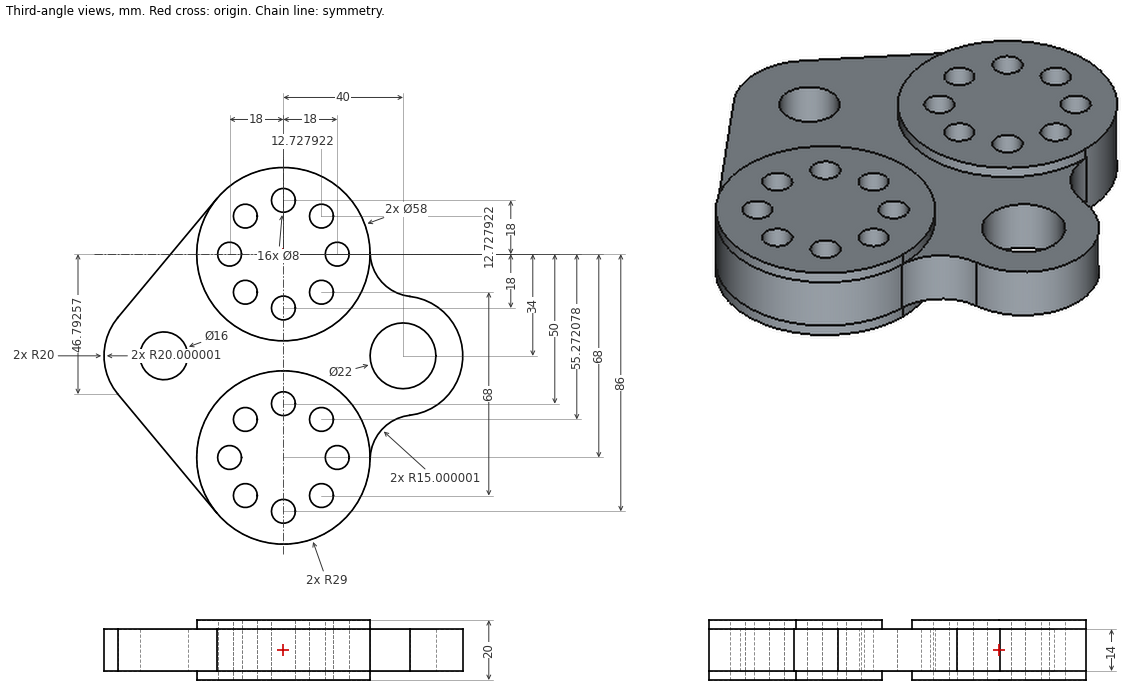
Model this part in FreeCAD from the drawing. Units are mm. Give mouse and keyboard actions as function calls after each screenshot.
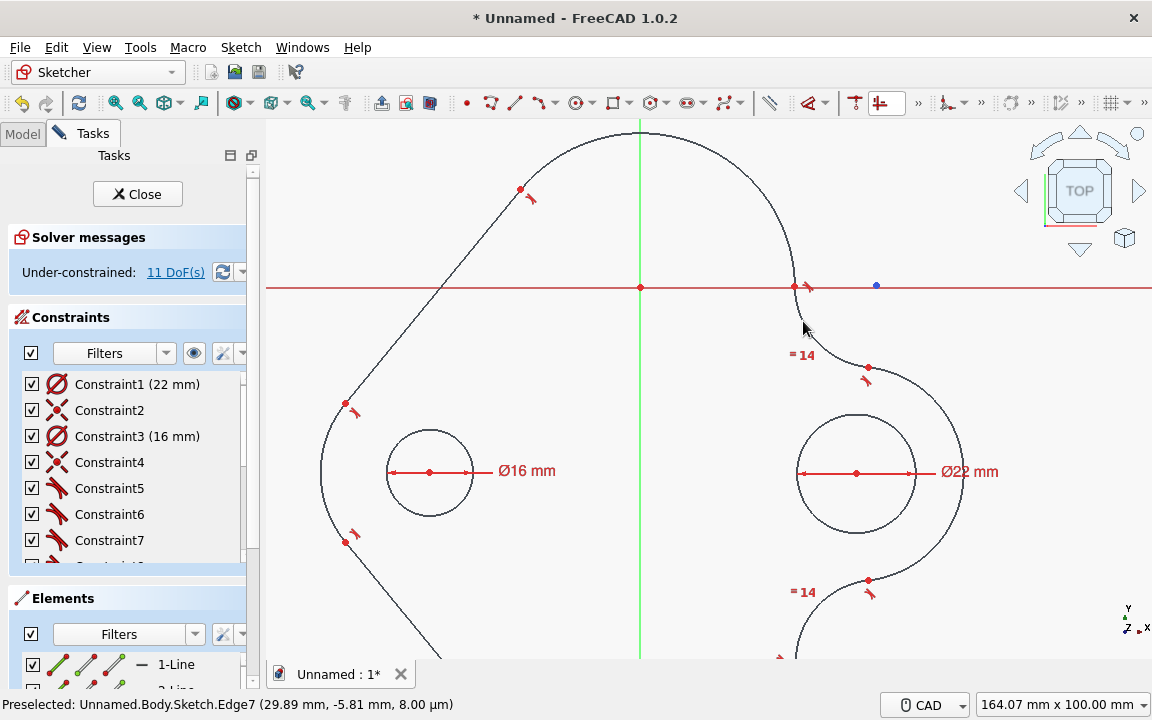
scroll(641, 289, down, 3)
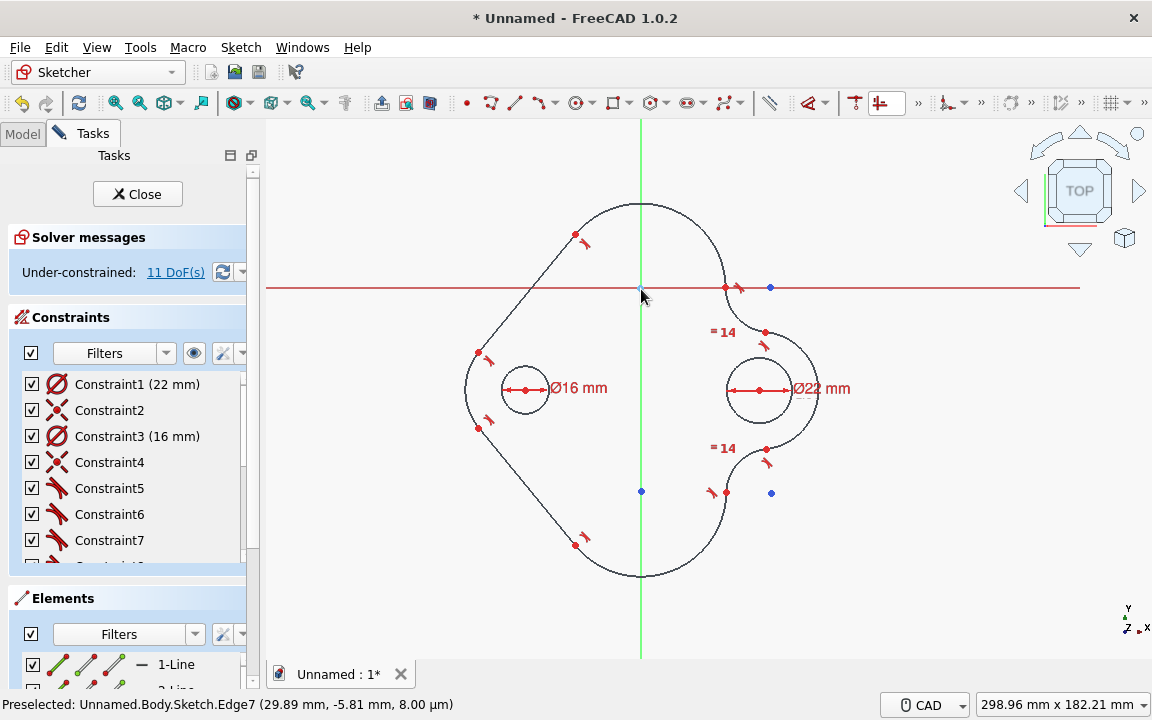
click(628, 576)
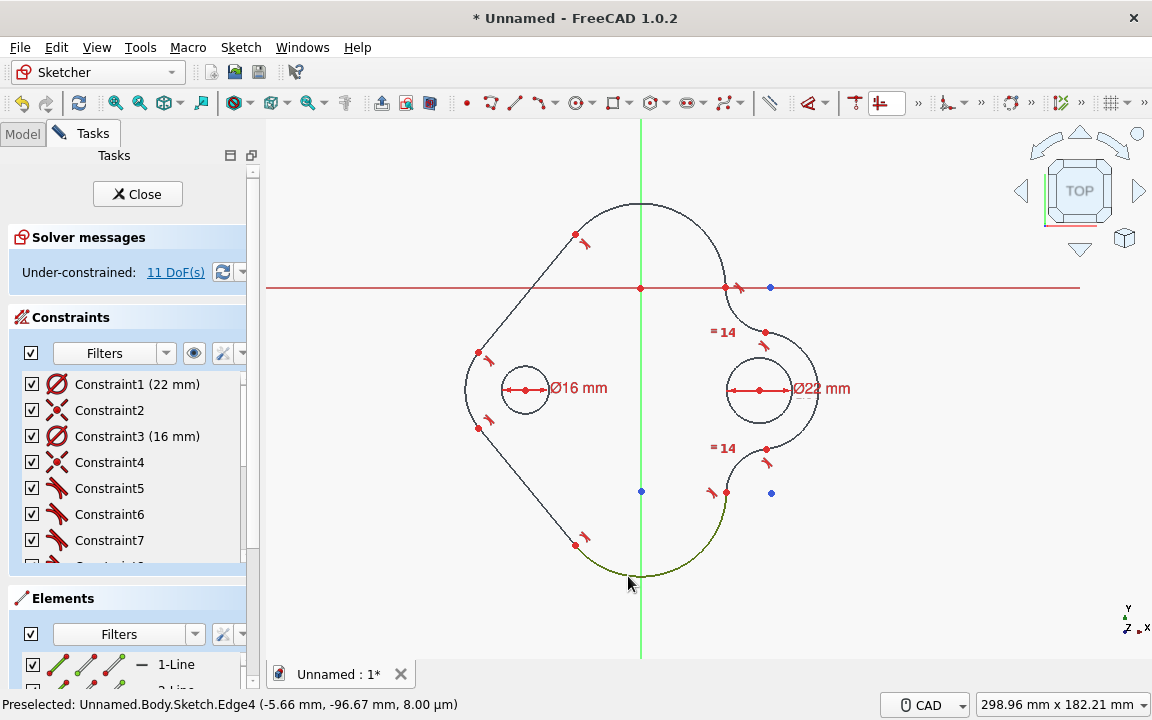
click(703, 231)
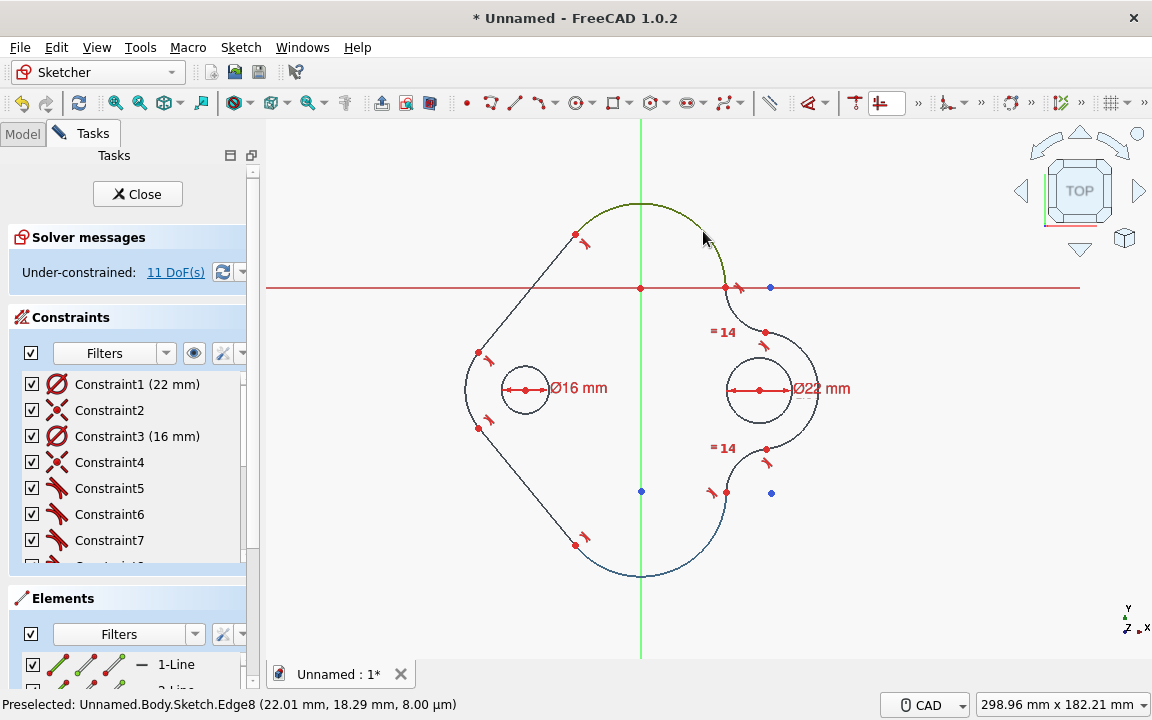
key(e)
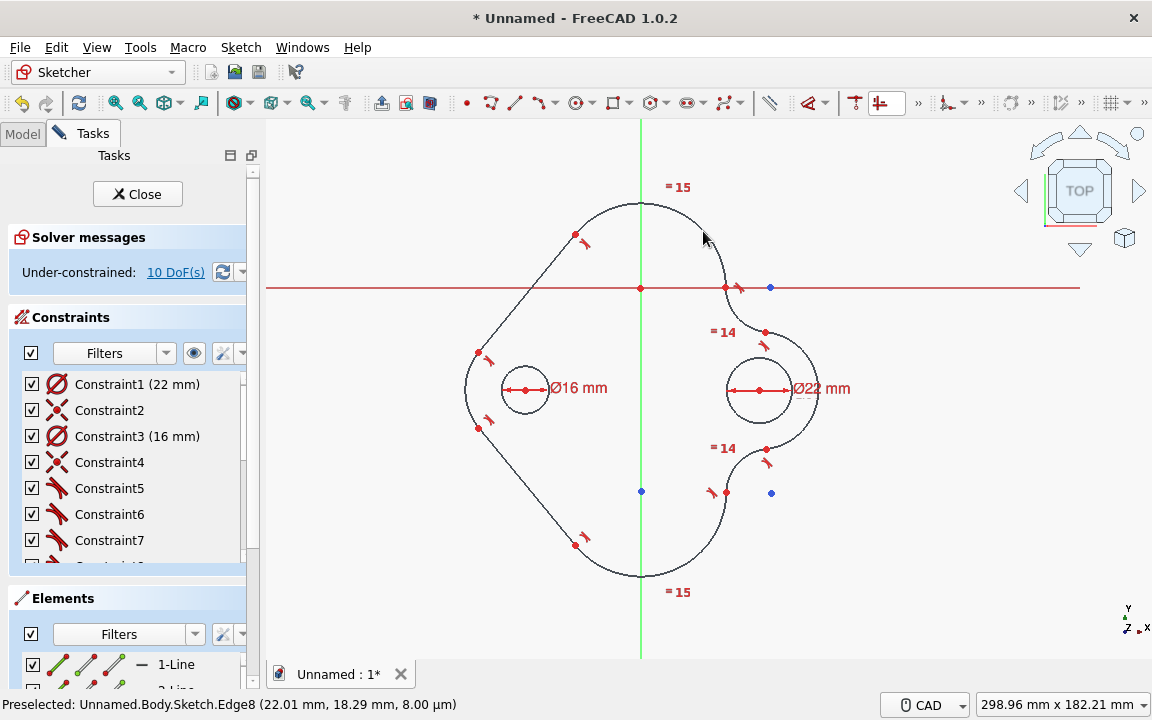
click(641, 492)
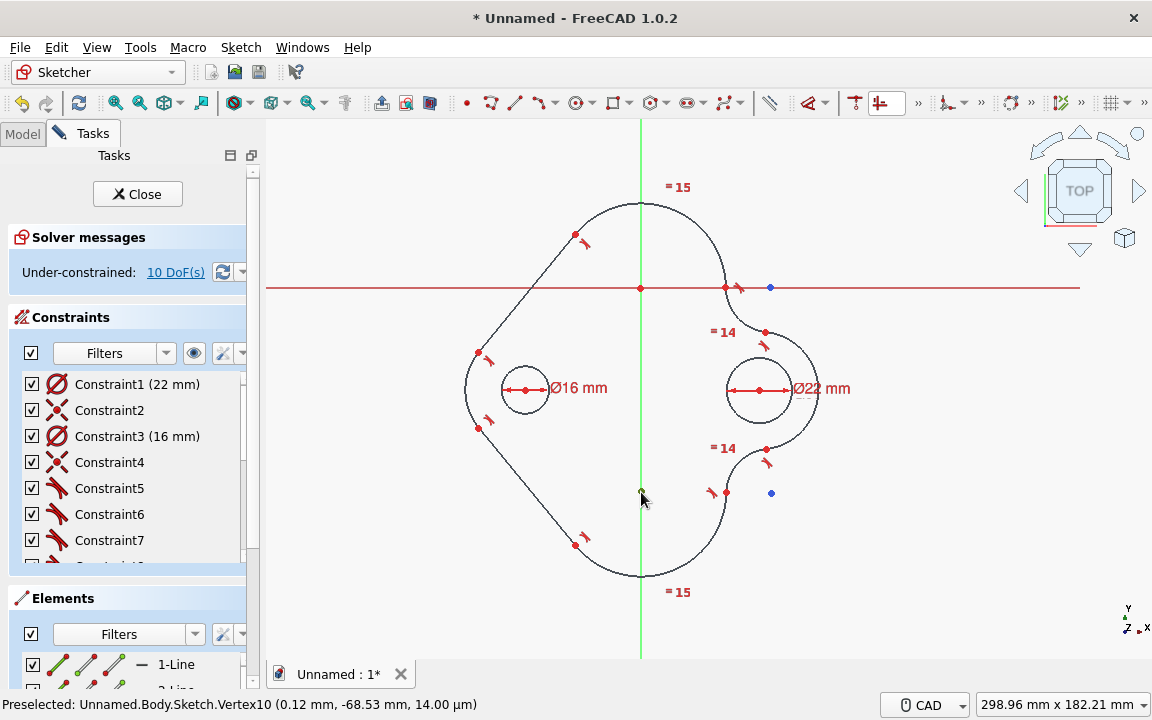
click(641, 527)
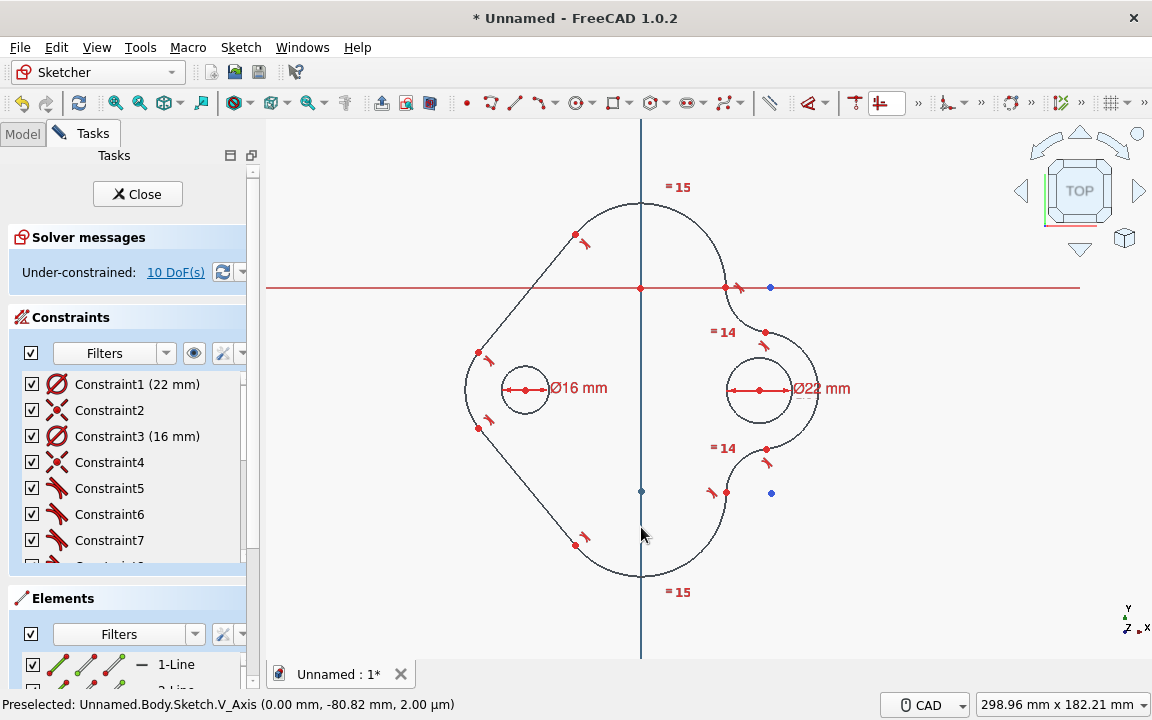
key(c)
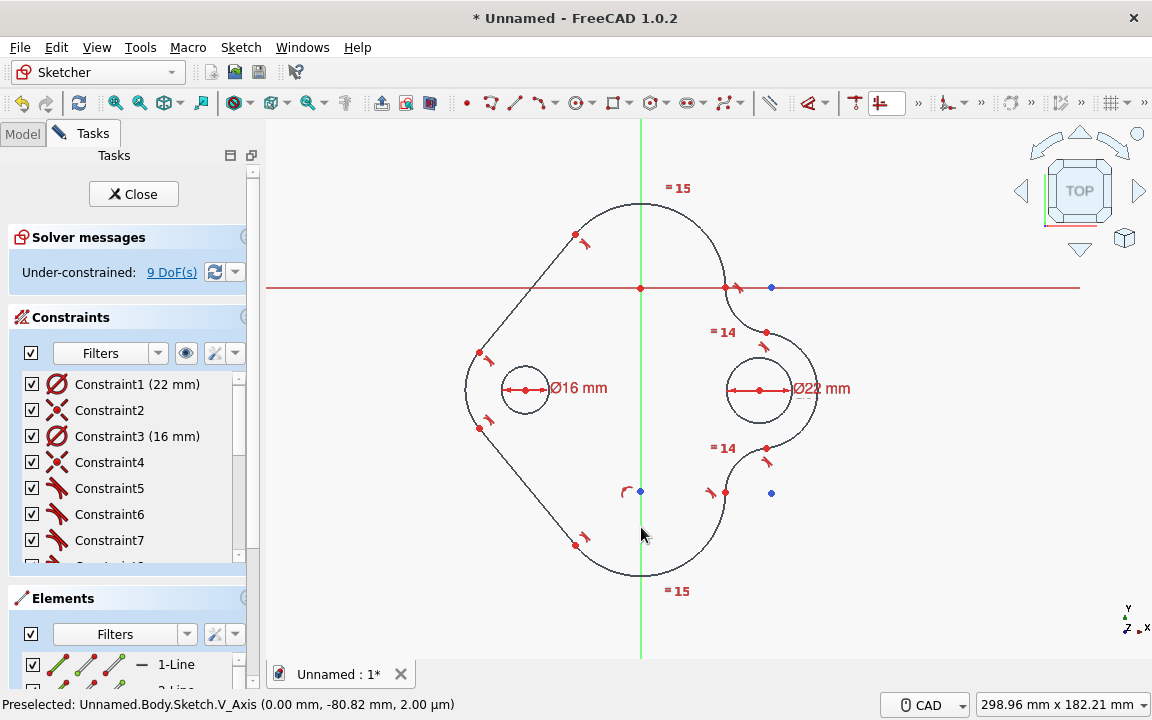
click(525, 390)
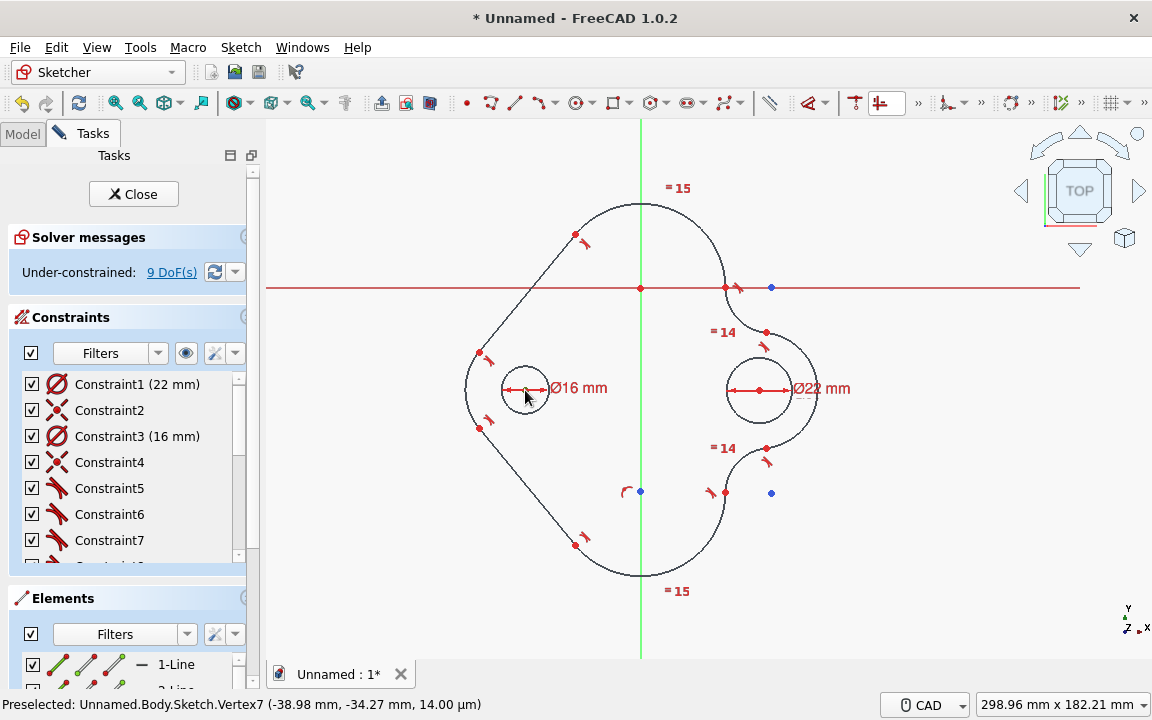
click(759, 391)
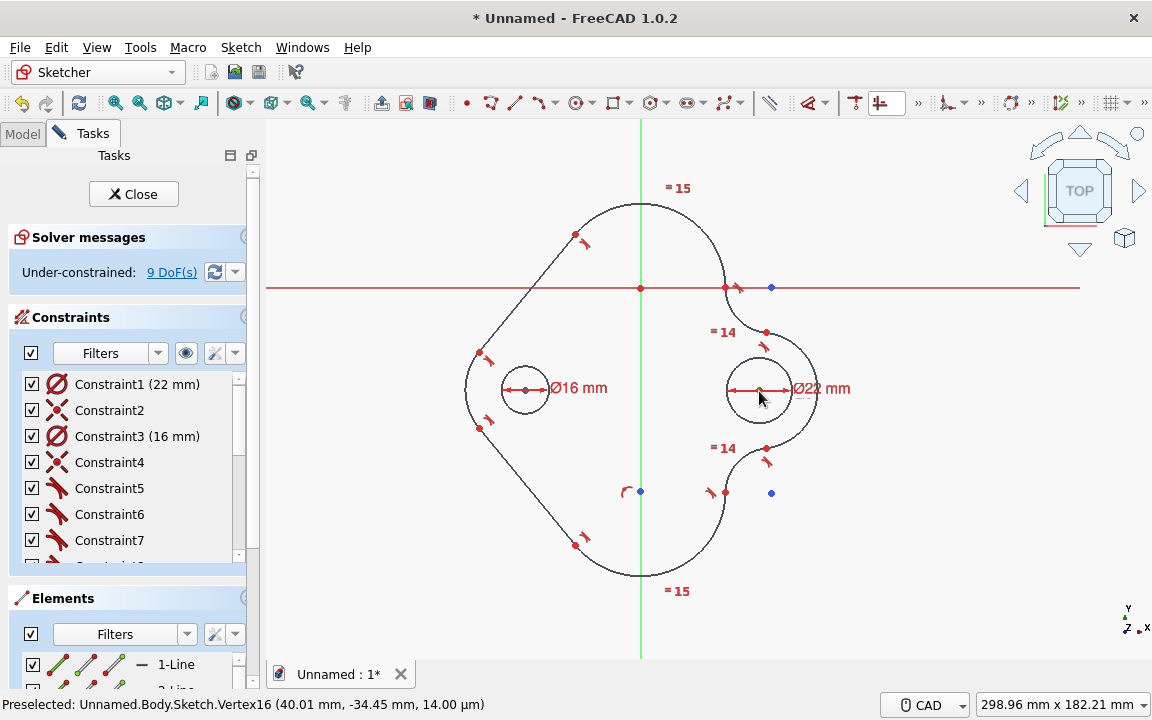
click(641, 527)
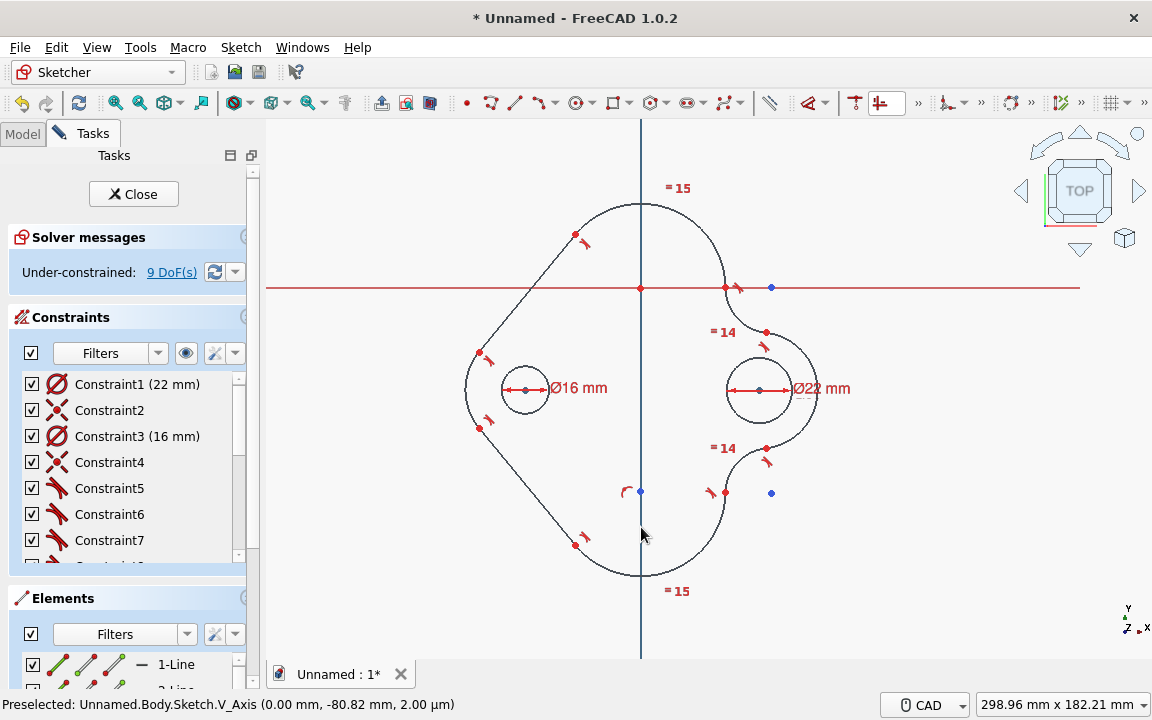
key(s)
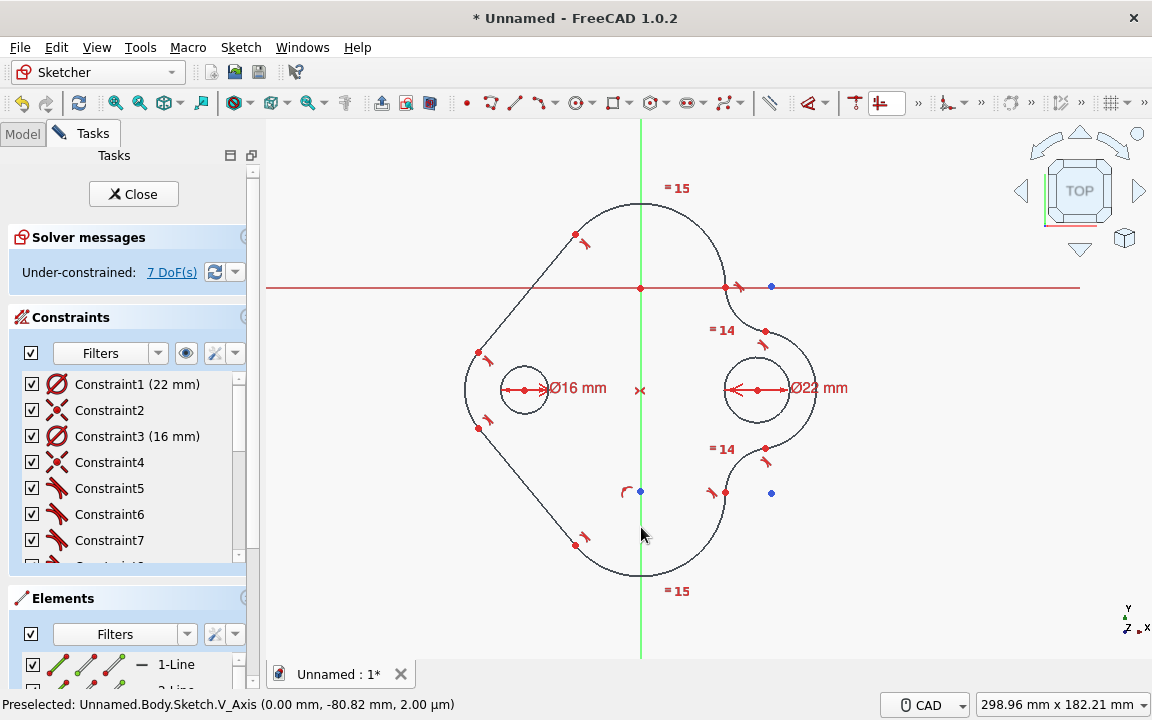
click(467, 374)